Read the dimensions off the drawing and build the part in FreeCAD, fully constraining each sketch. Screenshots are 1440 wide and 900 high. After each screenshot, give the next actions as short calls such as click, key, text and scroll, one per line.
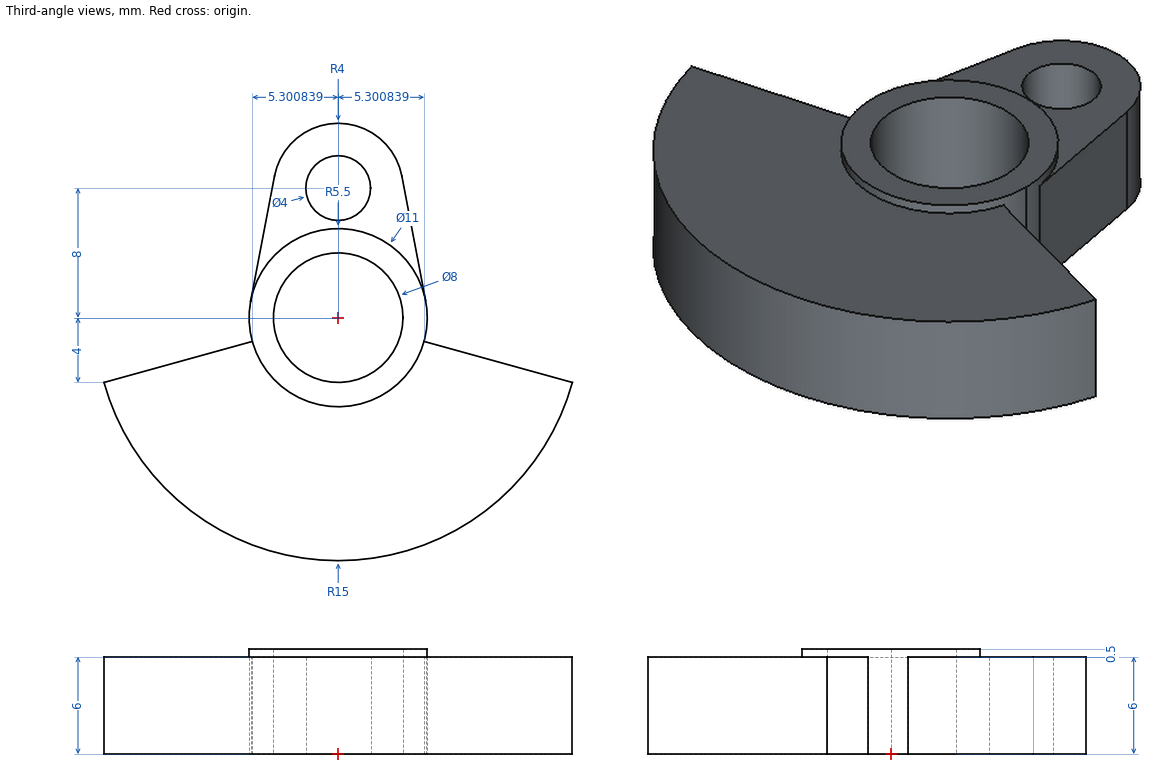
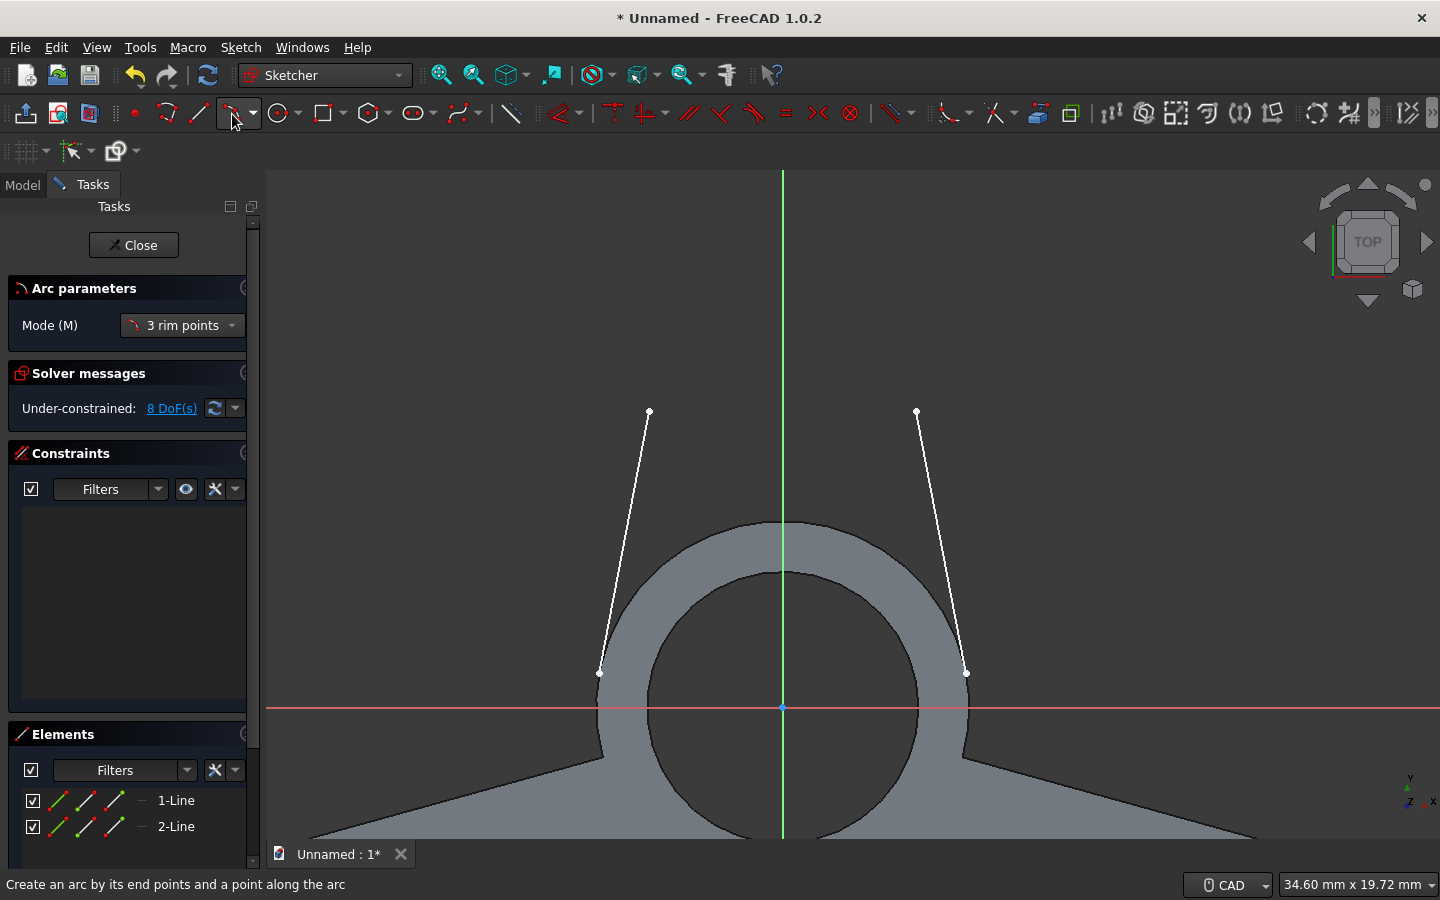
click(599, 674)
click(966, 674)
click(834, 528)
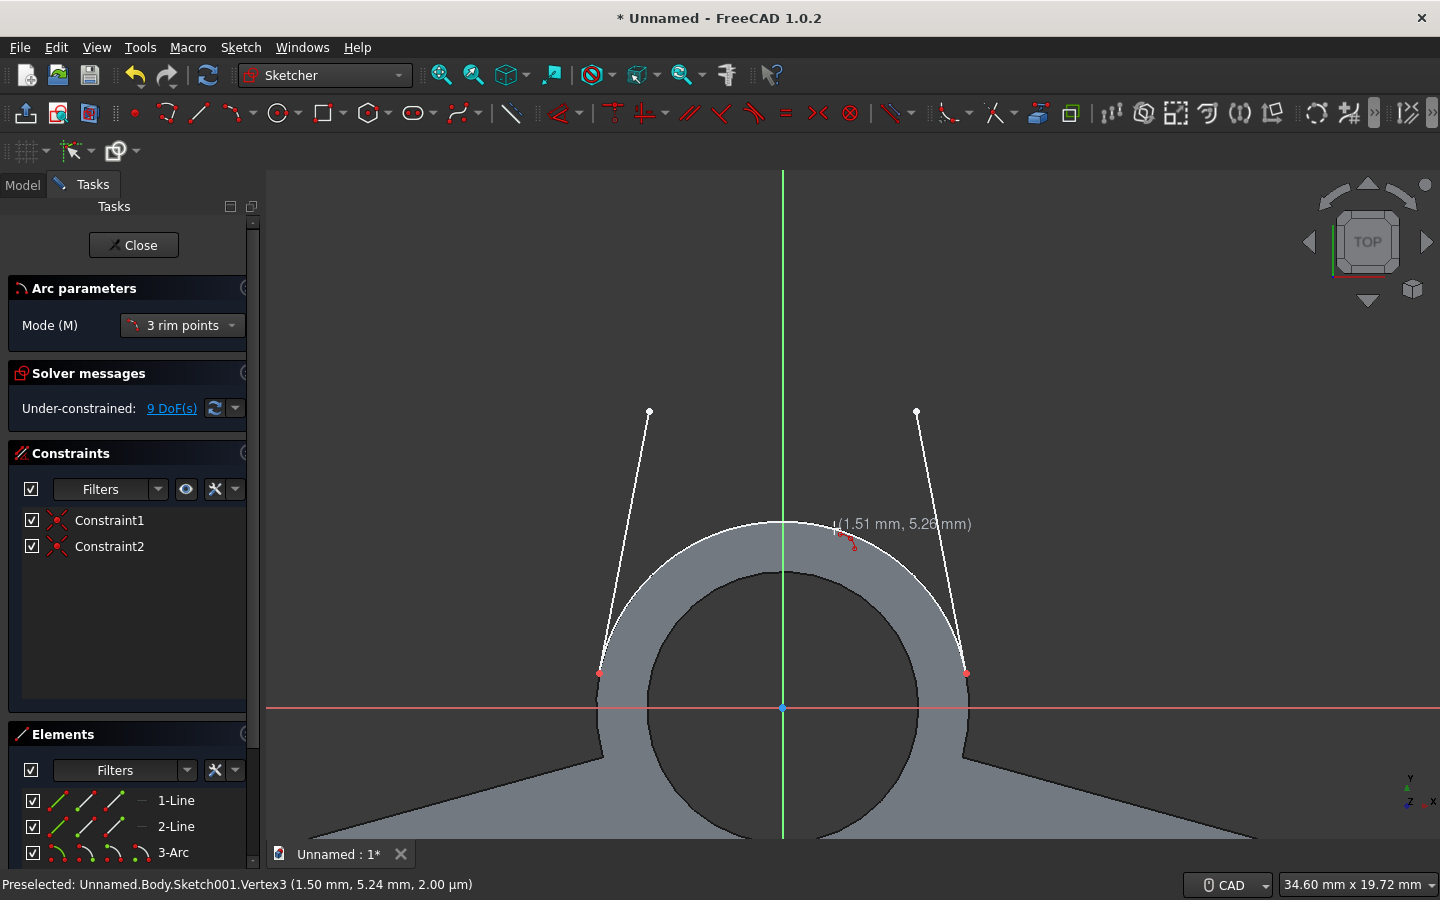
click(916, 412)
click(649, 412)
click(820, 306)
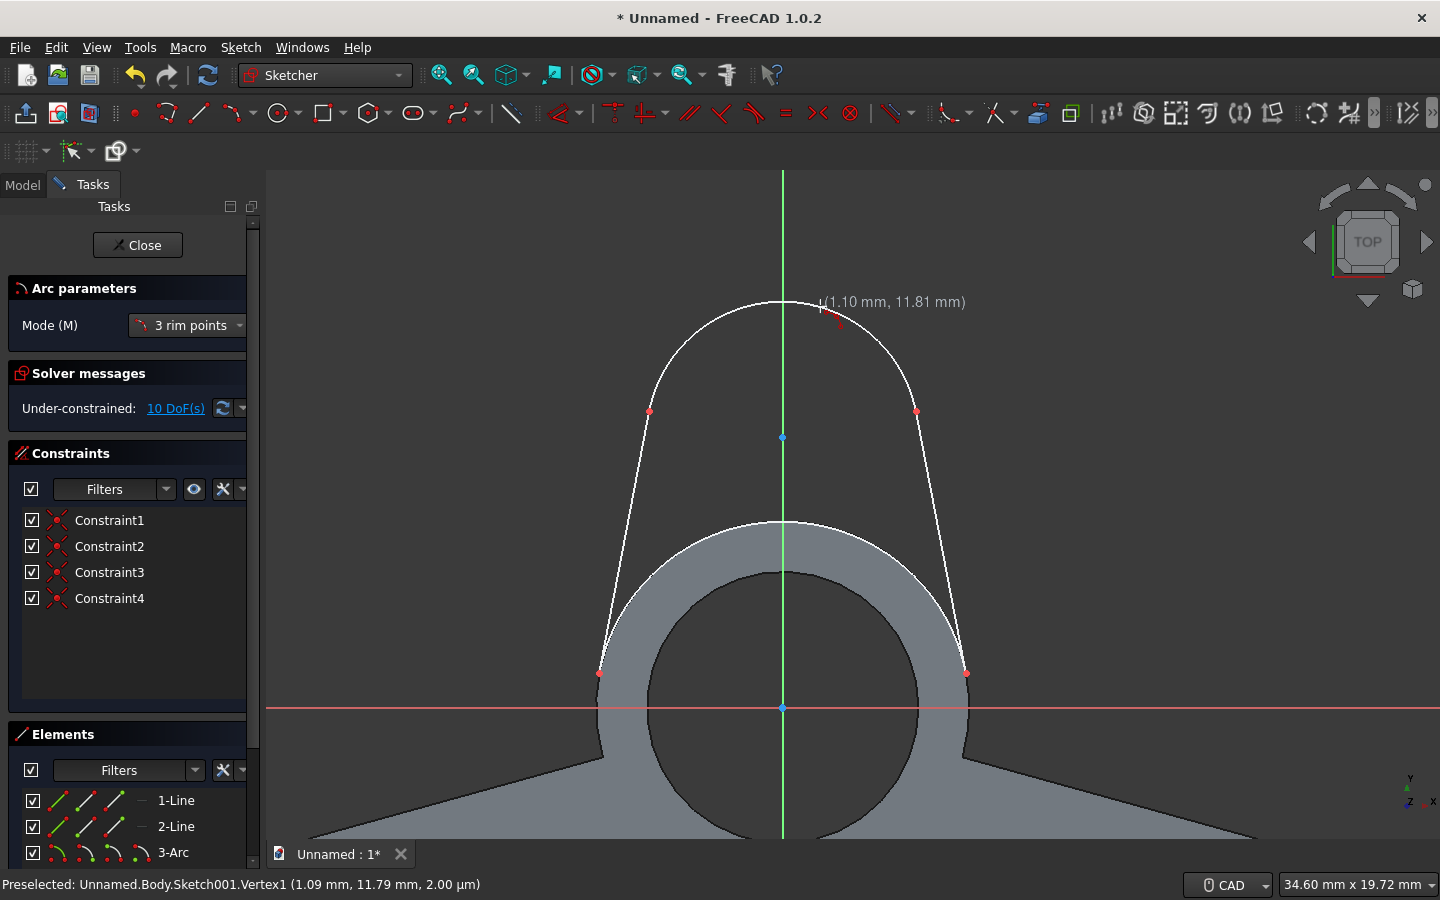
key(g)
key(c)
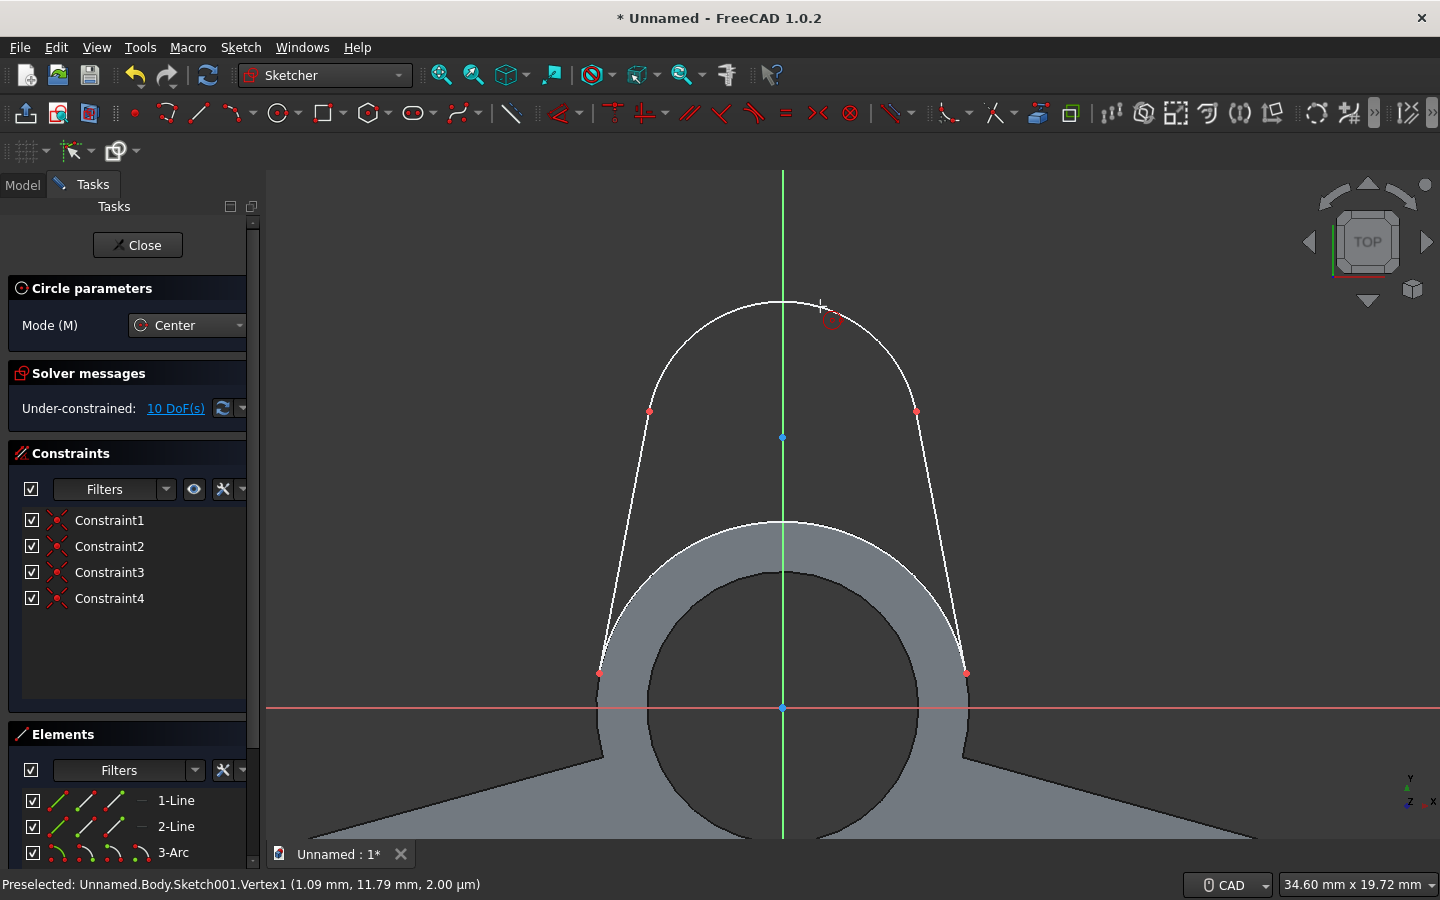
click(783, 436)
click(831, 388)
key(Escape)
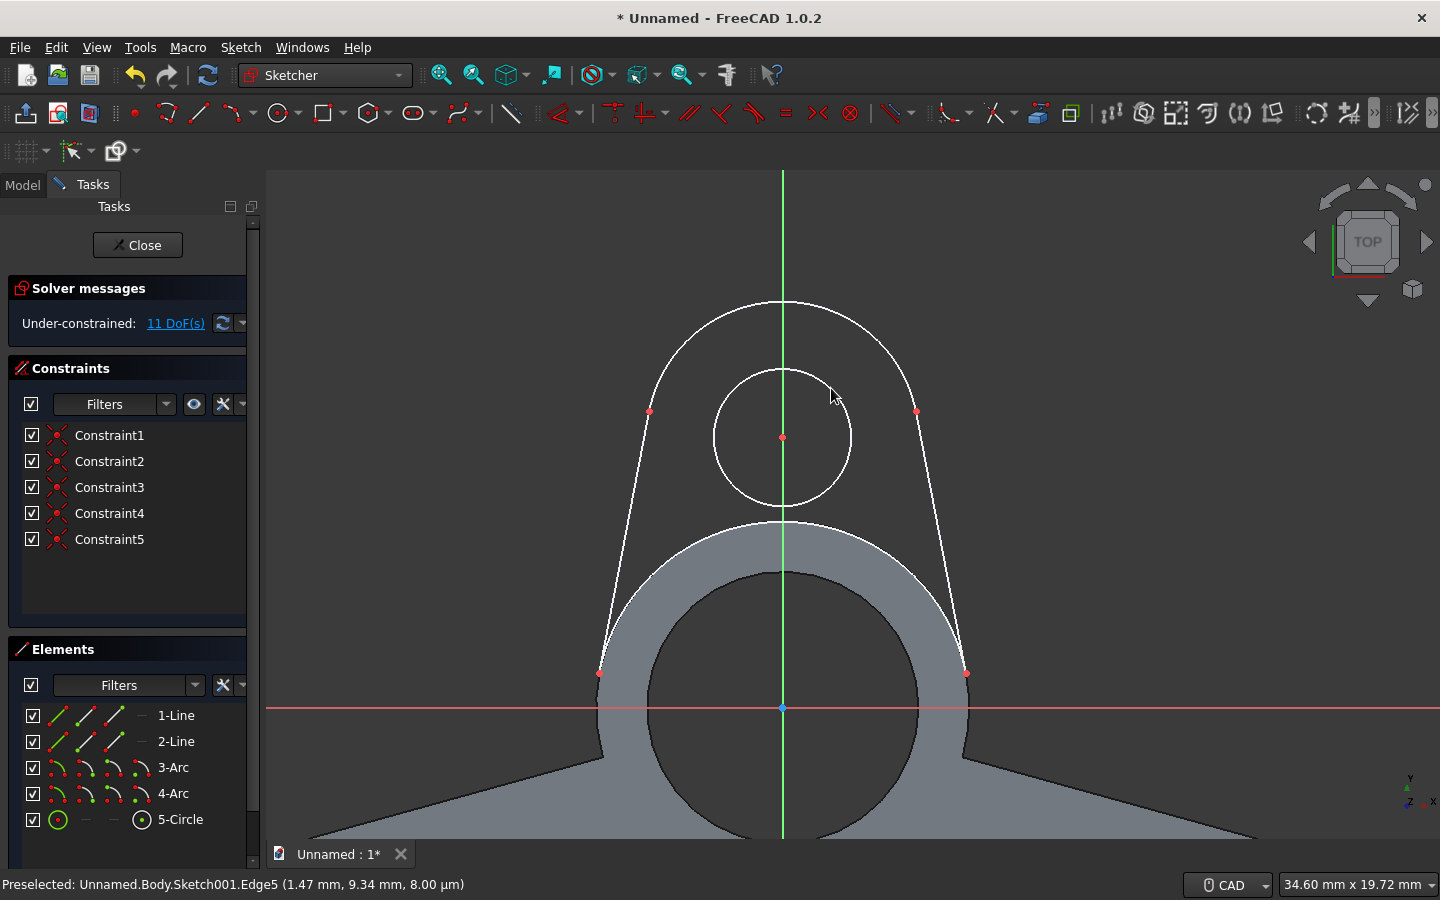
click(634, 491)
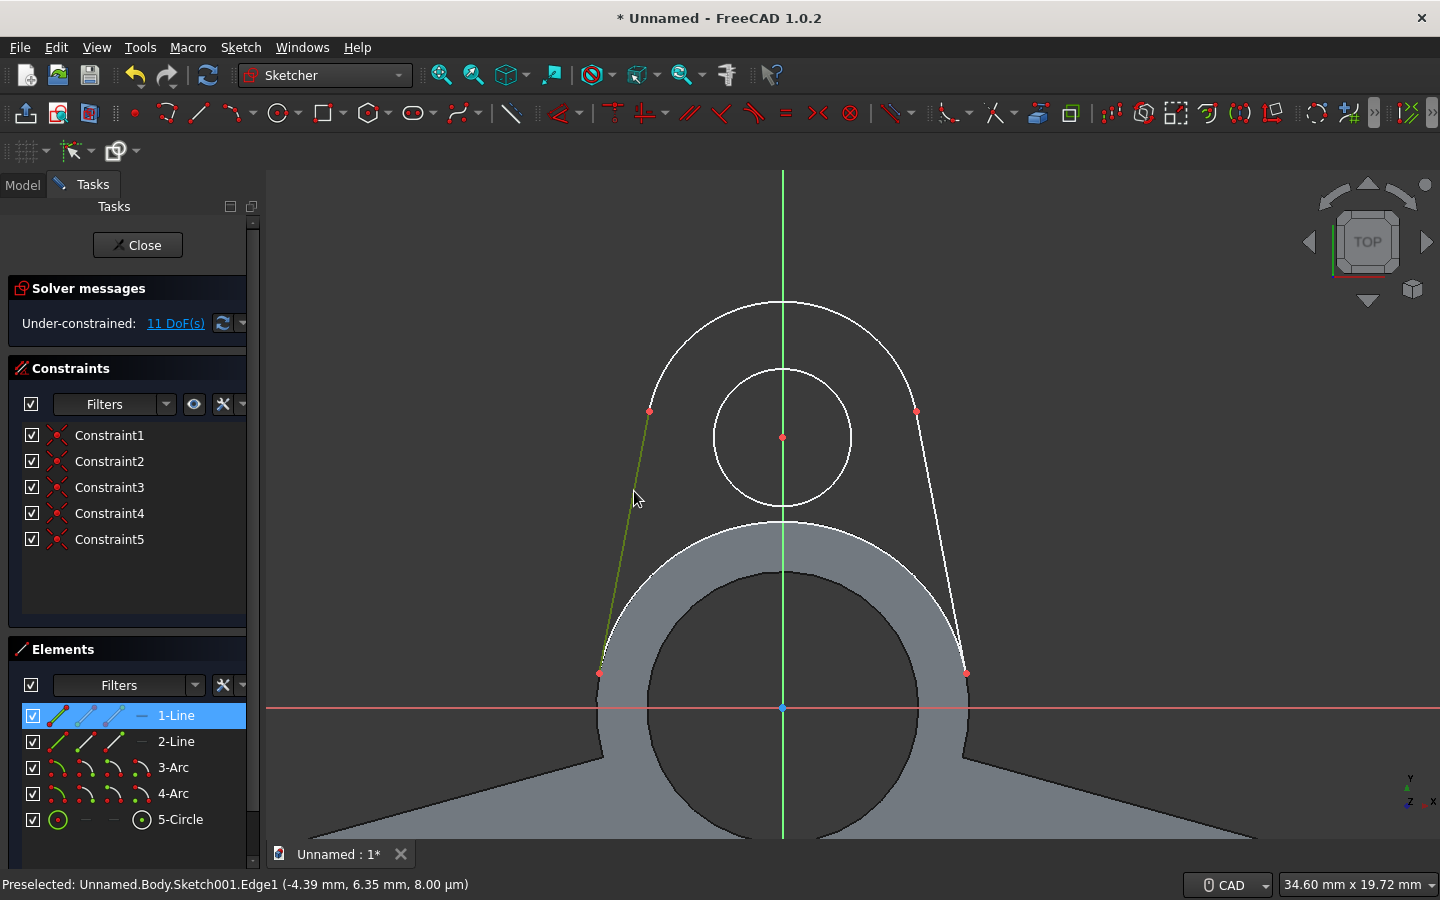
click(881, 550)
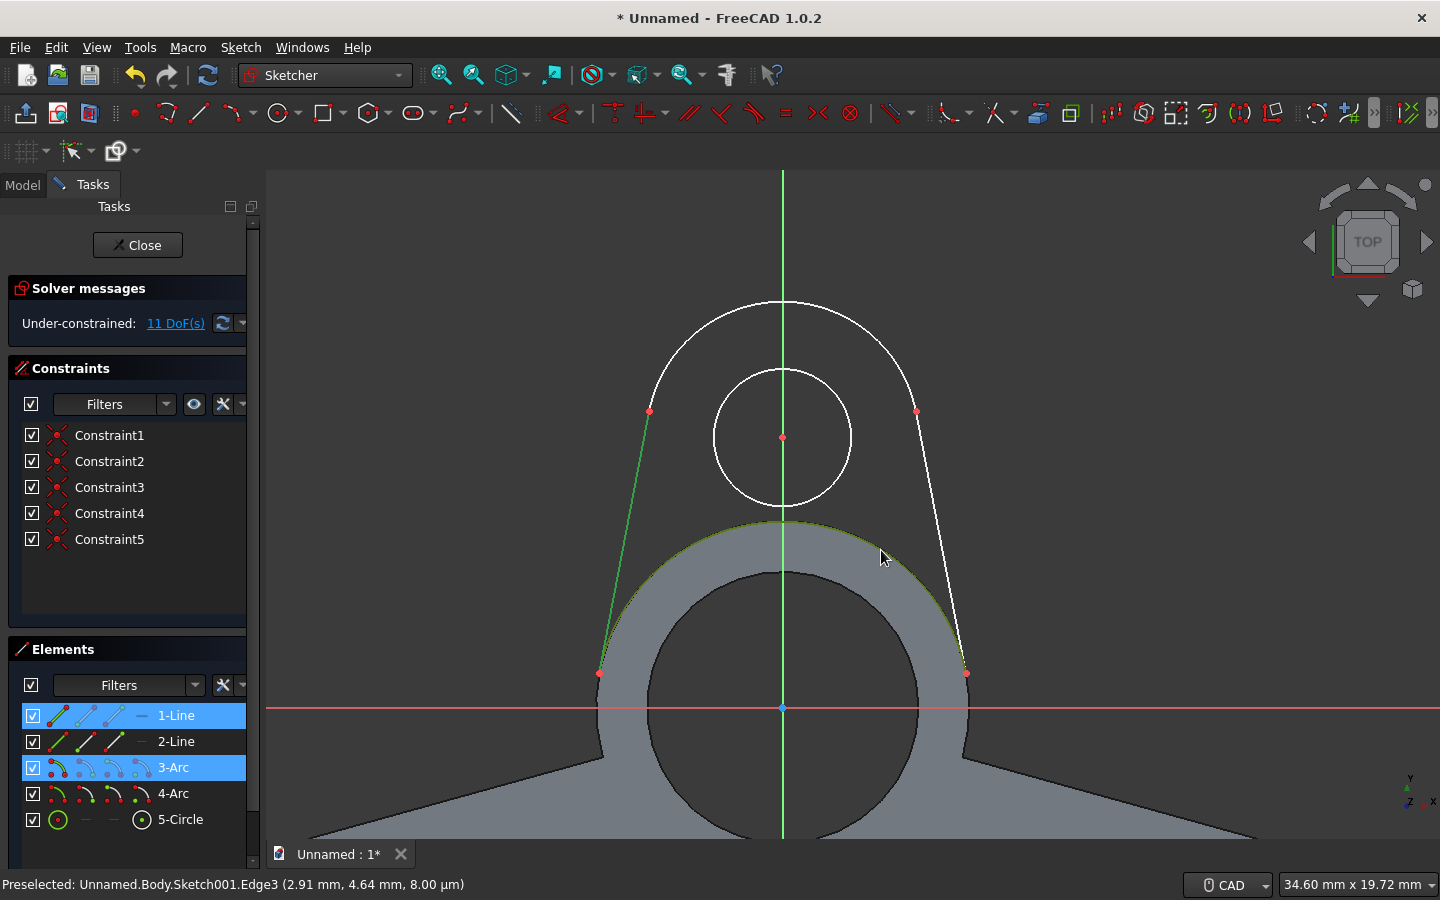
click(754, 114)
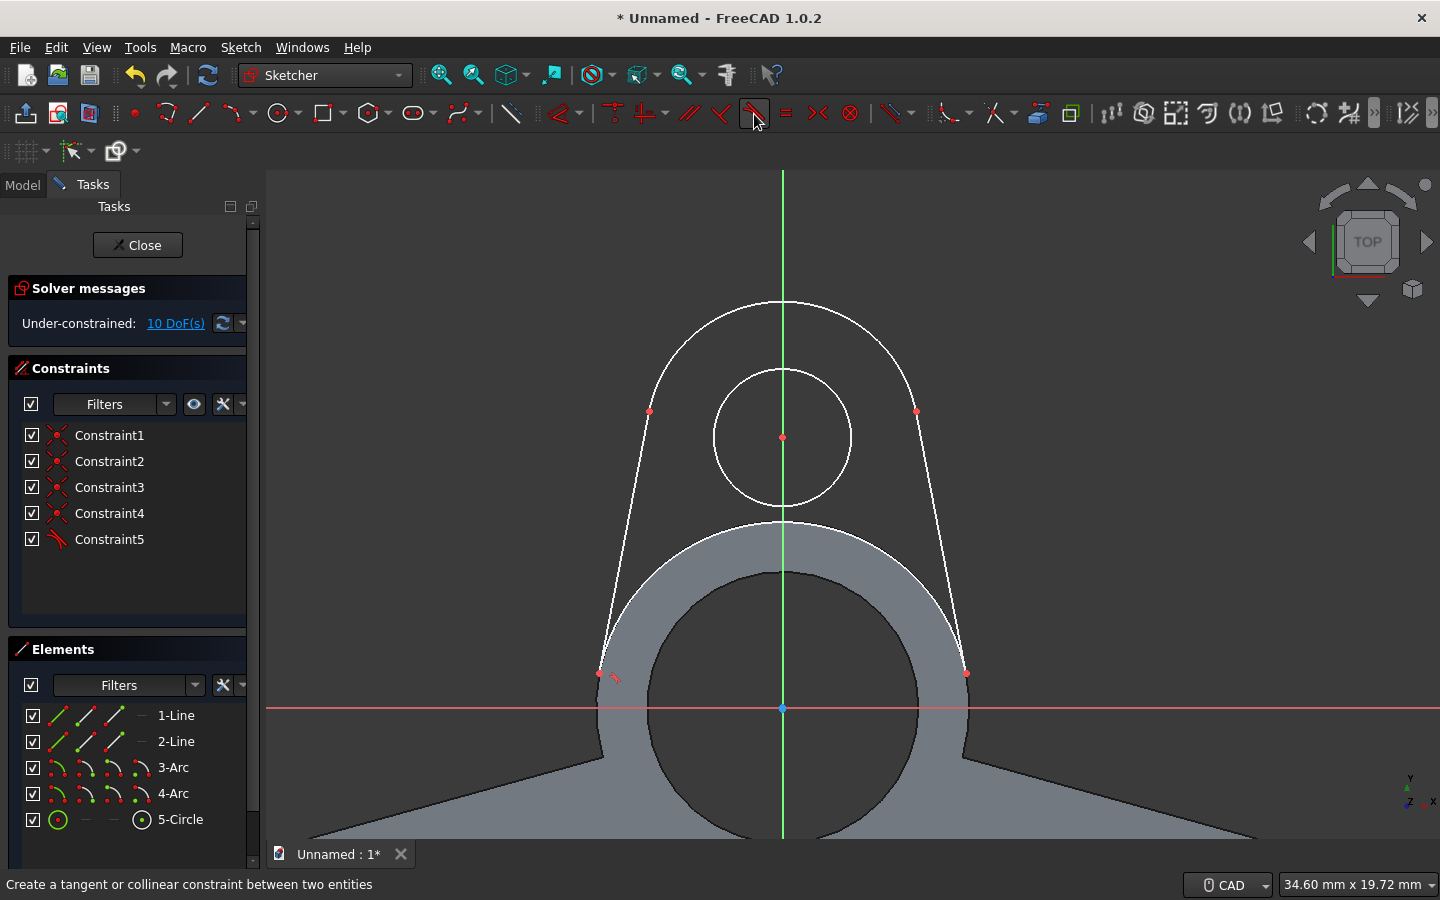
click(634, 491)